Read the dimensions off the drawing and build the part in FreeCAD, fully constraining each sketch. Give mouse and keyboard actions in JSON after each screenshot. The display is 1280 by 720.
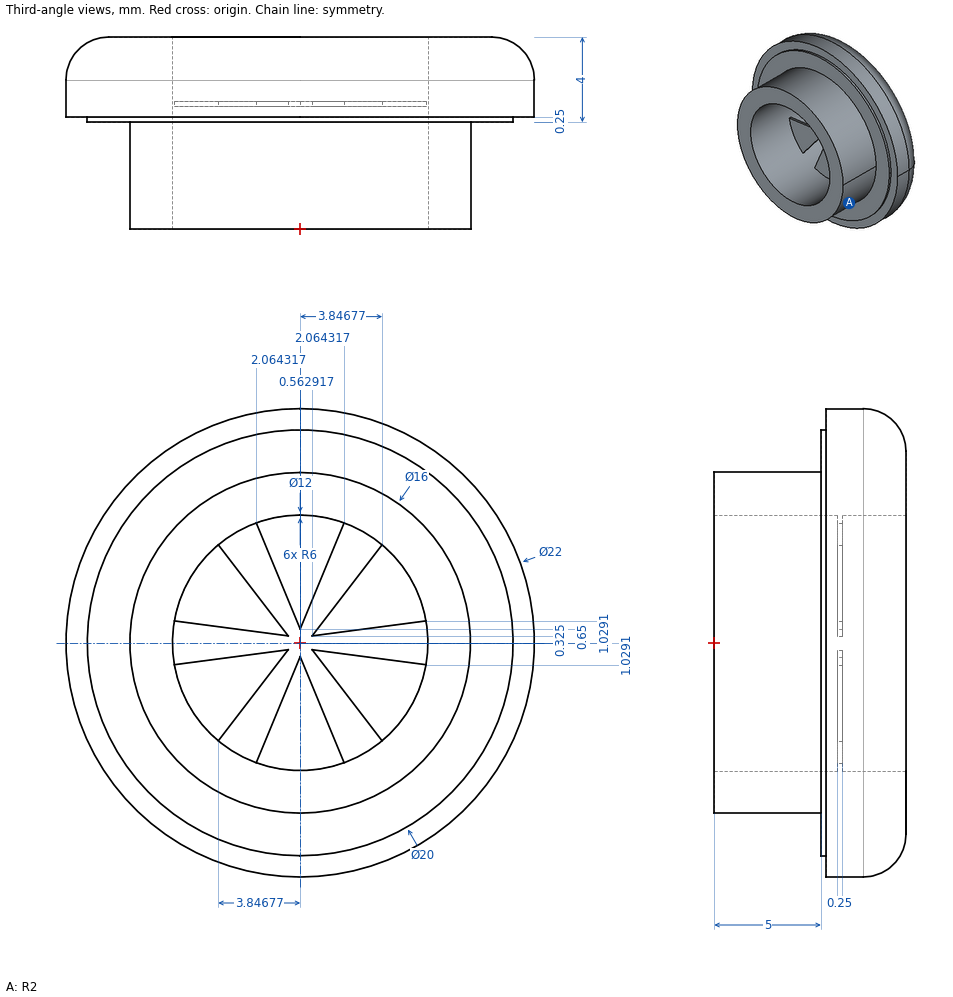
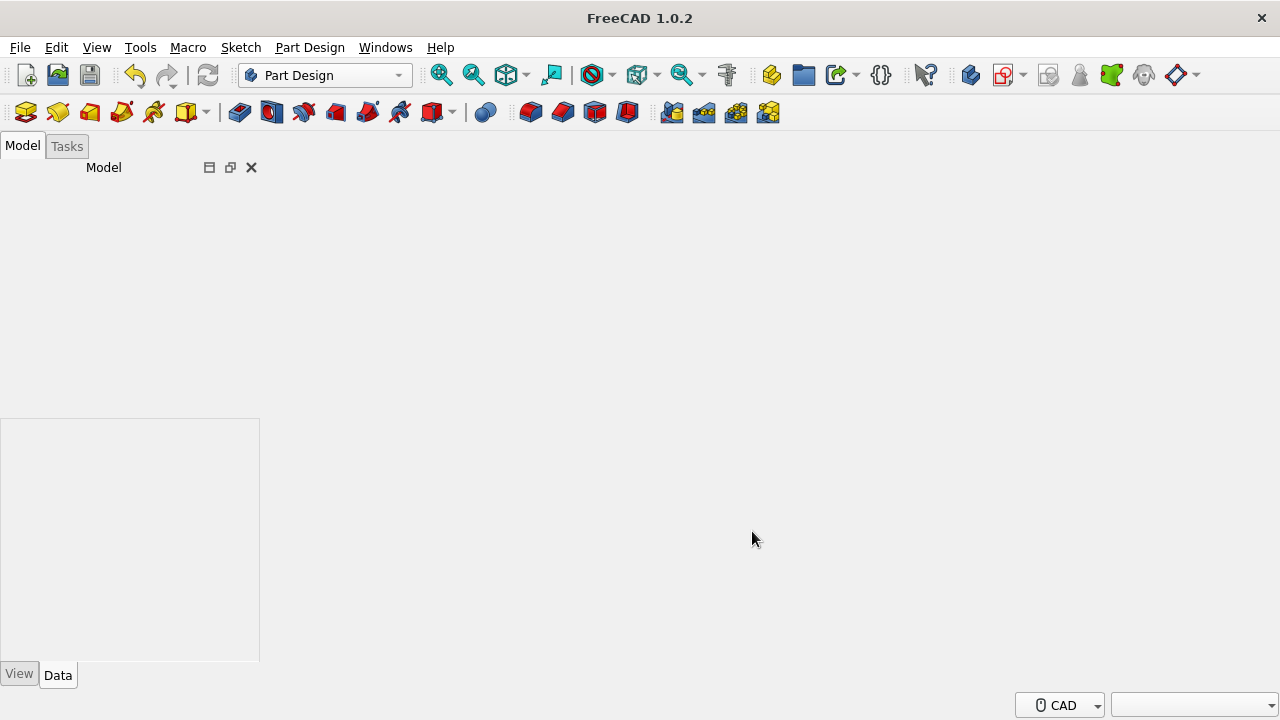
{"action": "key", "text": "ctrl+n"}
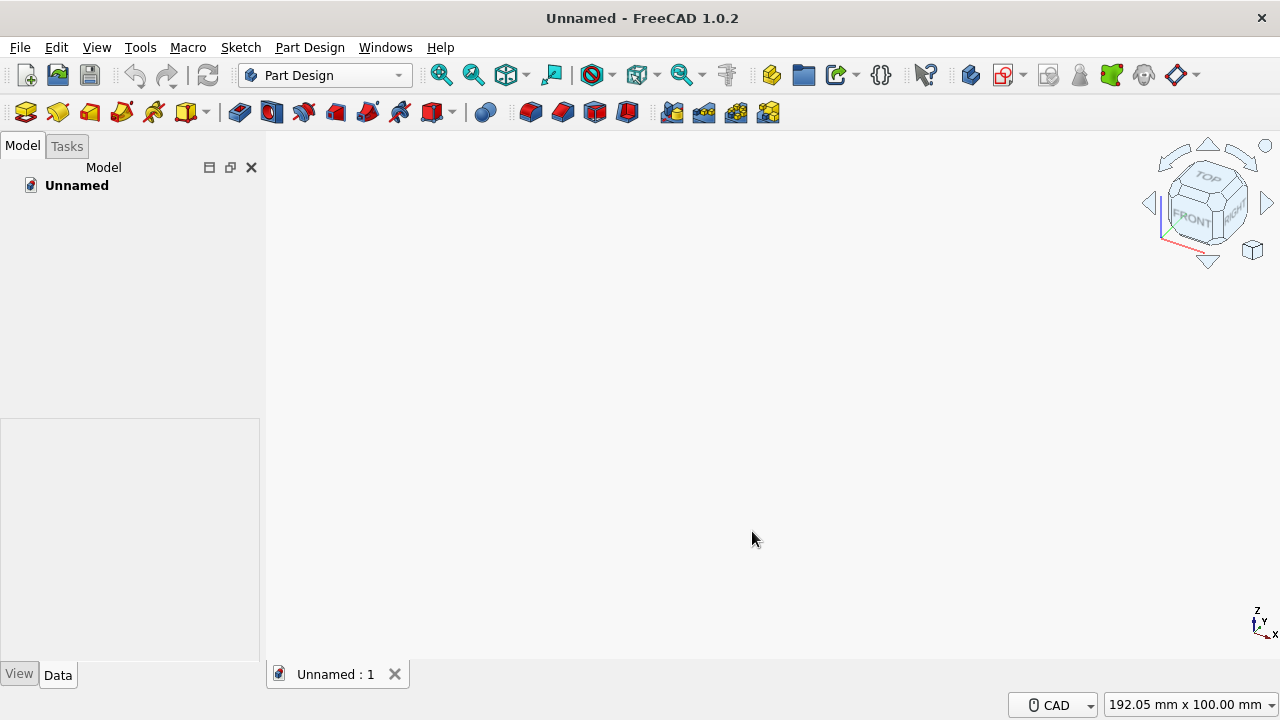
{"action": "left_click", "coordinate": [1004, 76]}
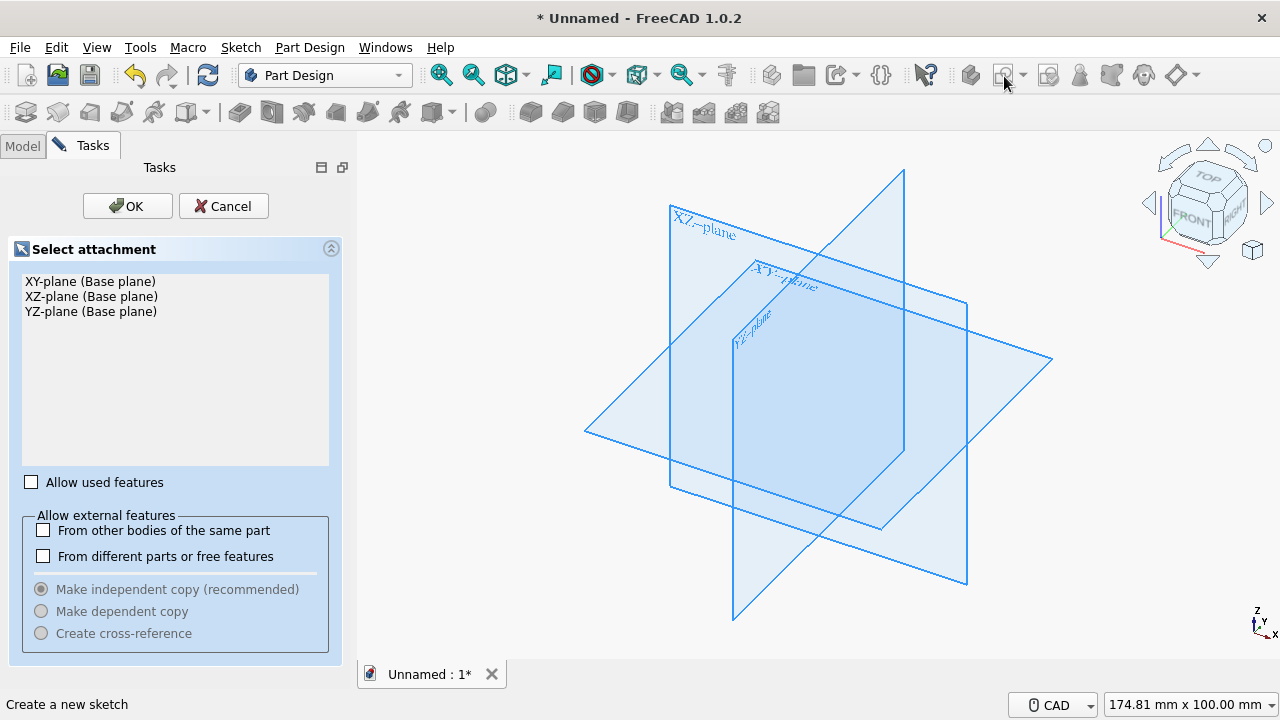
{"action": "left_click", "coordinate": [82, 296]}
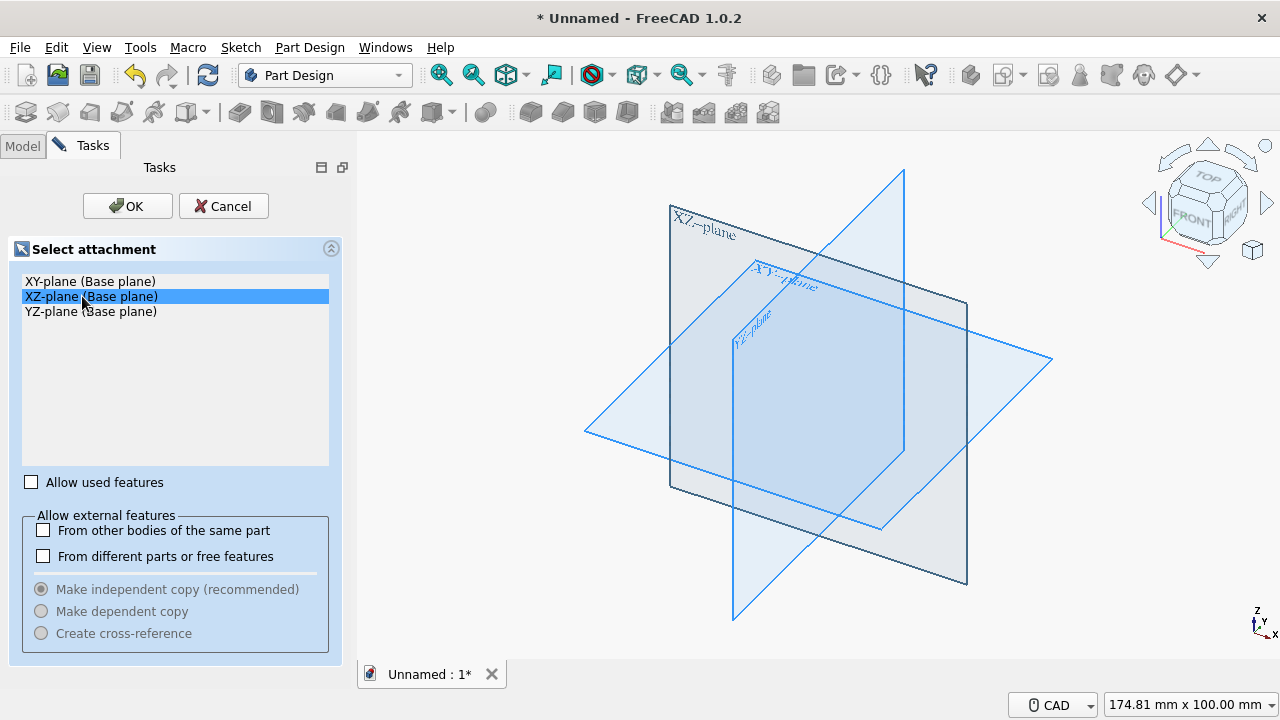
{"action": "left_click", "coordinate": [128, 206]}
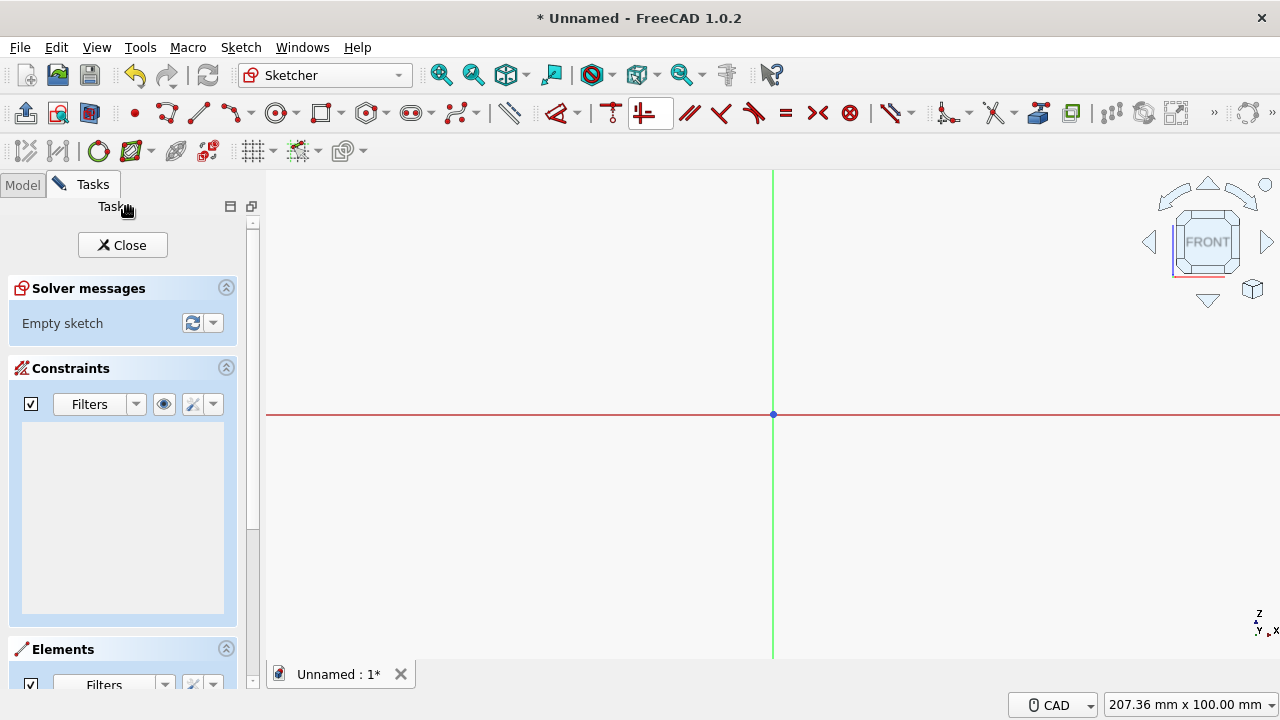
{"action": "scroll", "coordinate": [795, 415], "scroll_direction": "up", "scroll_amount": 7}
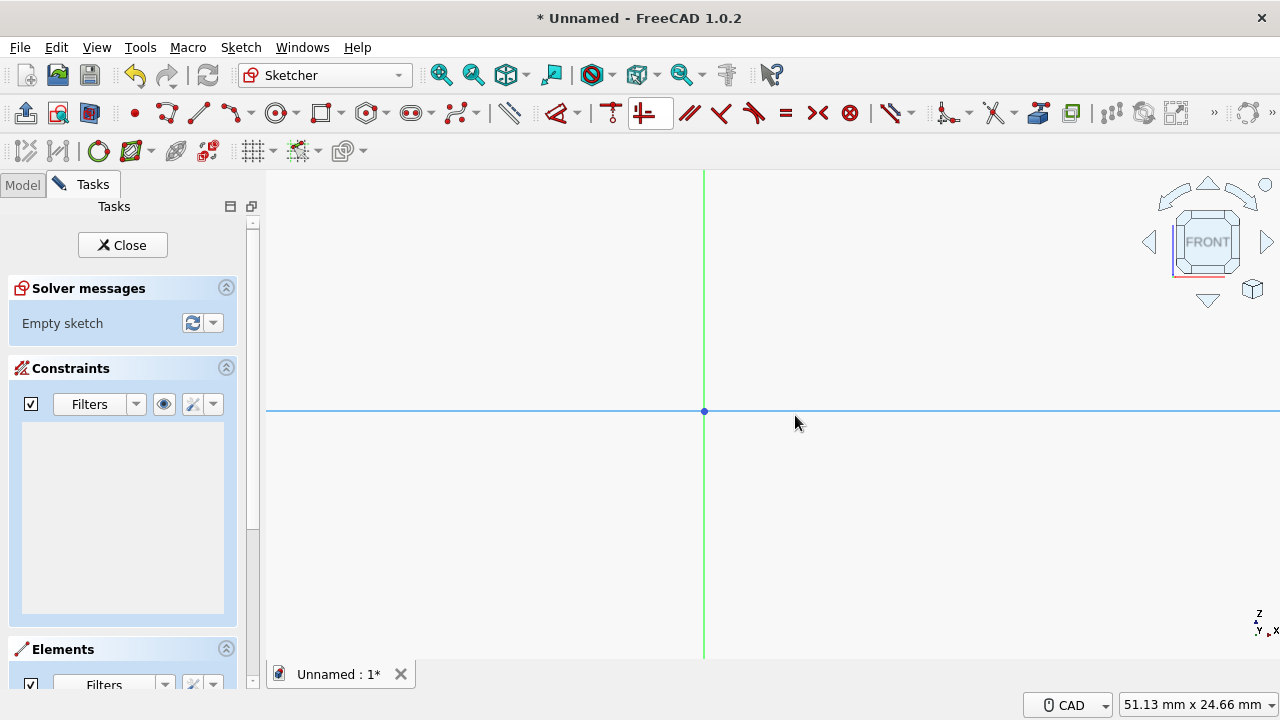
{"action": "key", "text": "g c"}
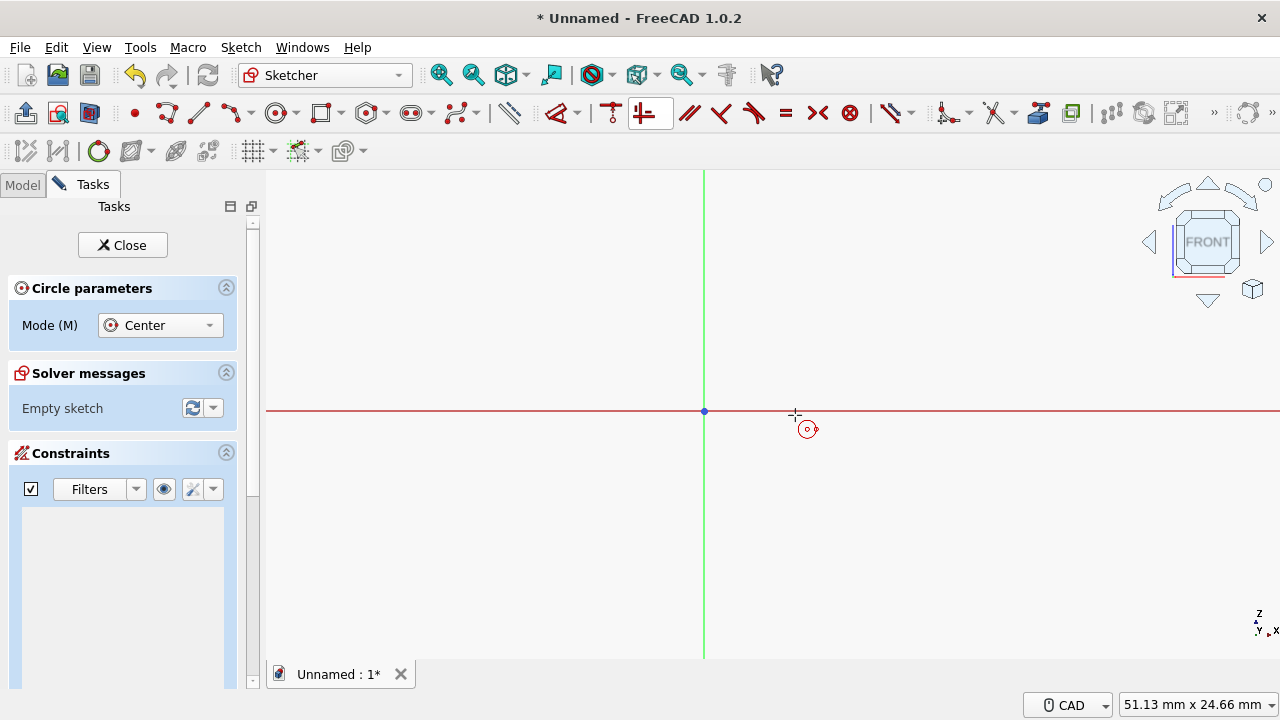
{"action": "left_click", "coordinate": [704, 411]}
{"action": "left_click", "coordinate": [816, 299]}
{"action": "key", "text": "Escape"}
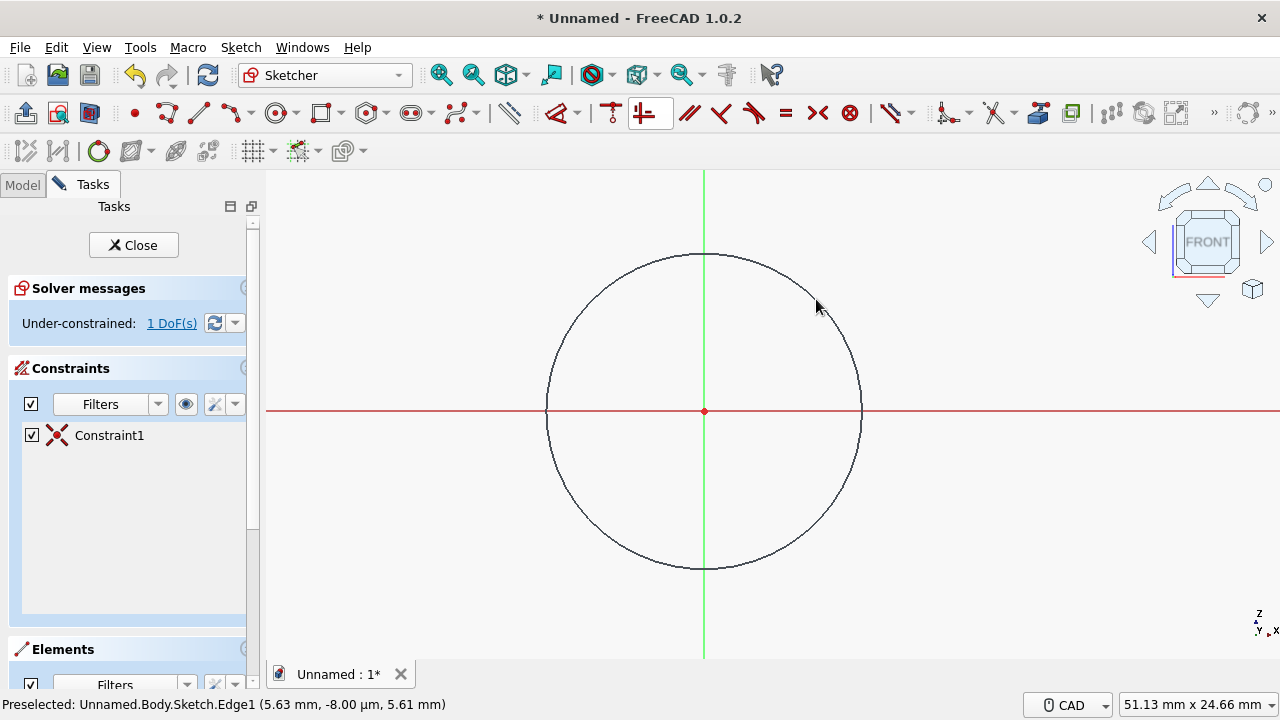
{"action": "key", "text": "d"}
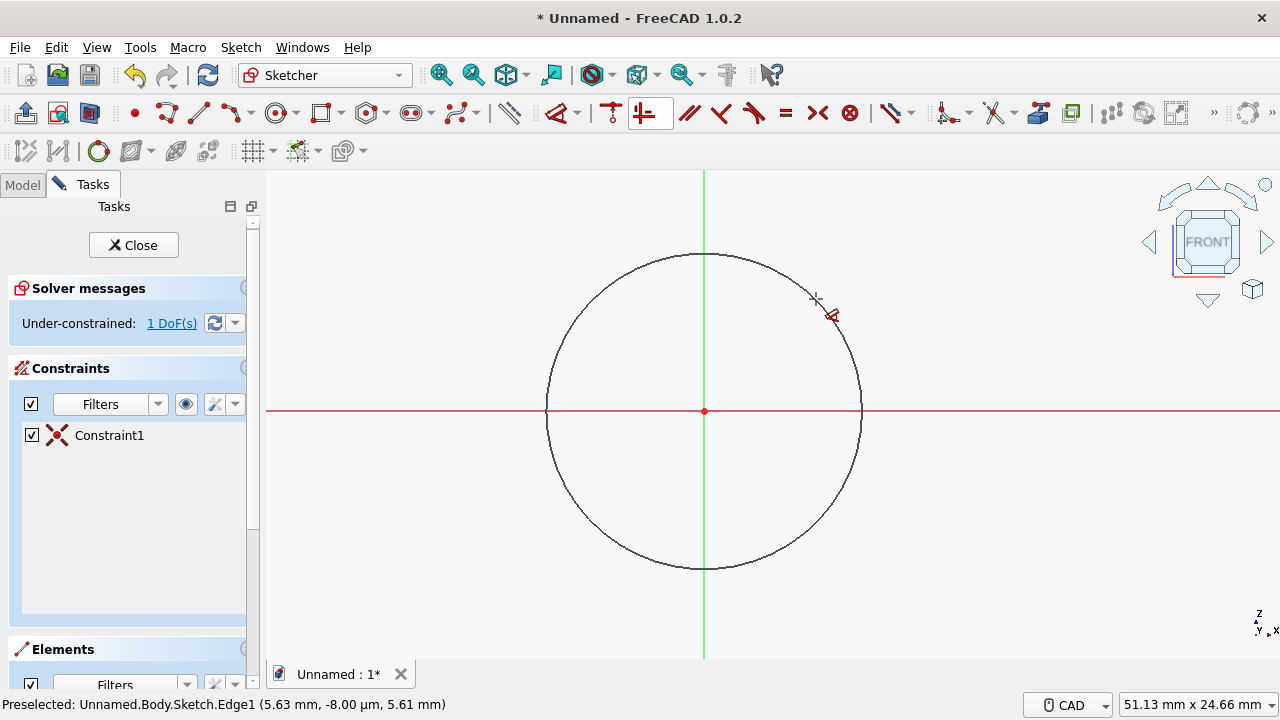
{"action": "left_click", "coordinate": [815, 299]}
{"action": "left_click", "coordinate": [837, 276]}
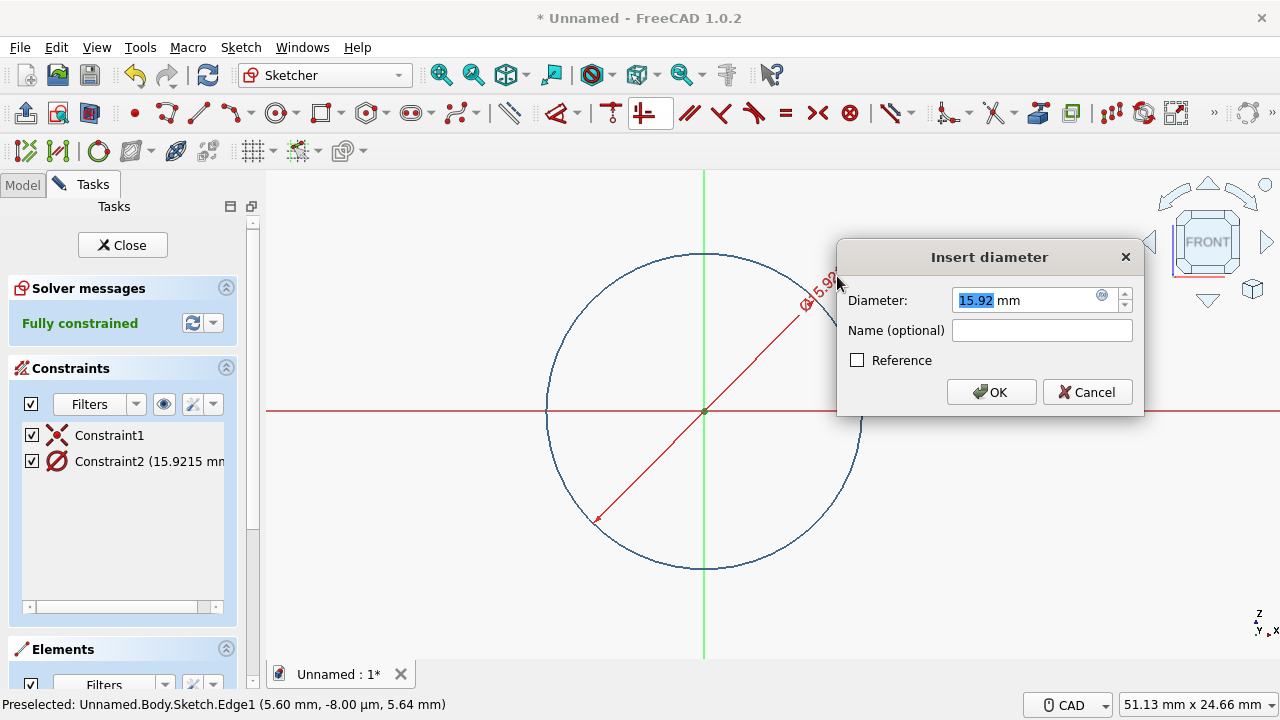
{"action": "type", "text": "16"}
{"action": "key", "text": "Return"}
{"action": "key", "text": "Escape"}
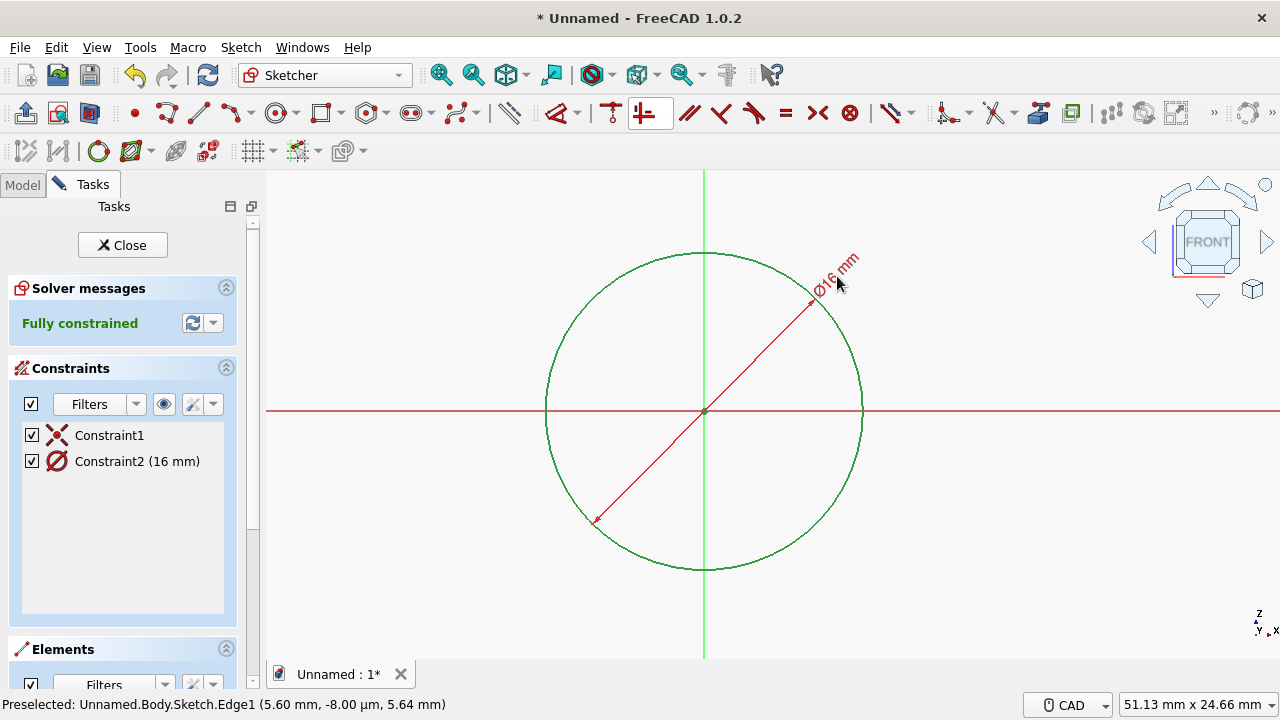
{"action": "left_click", "coordinate": [123, 245]}